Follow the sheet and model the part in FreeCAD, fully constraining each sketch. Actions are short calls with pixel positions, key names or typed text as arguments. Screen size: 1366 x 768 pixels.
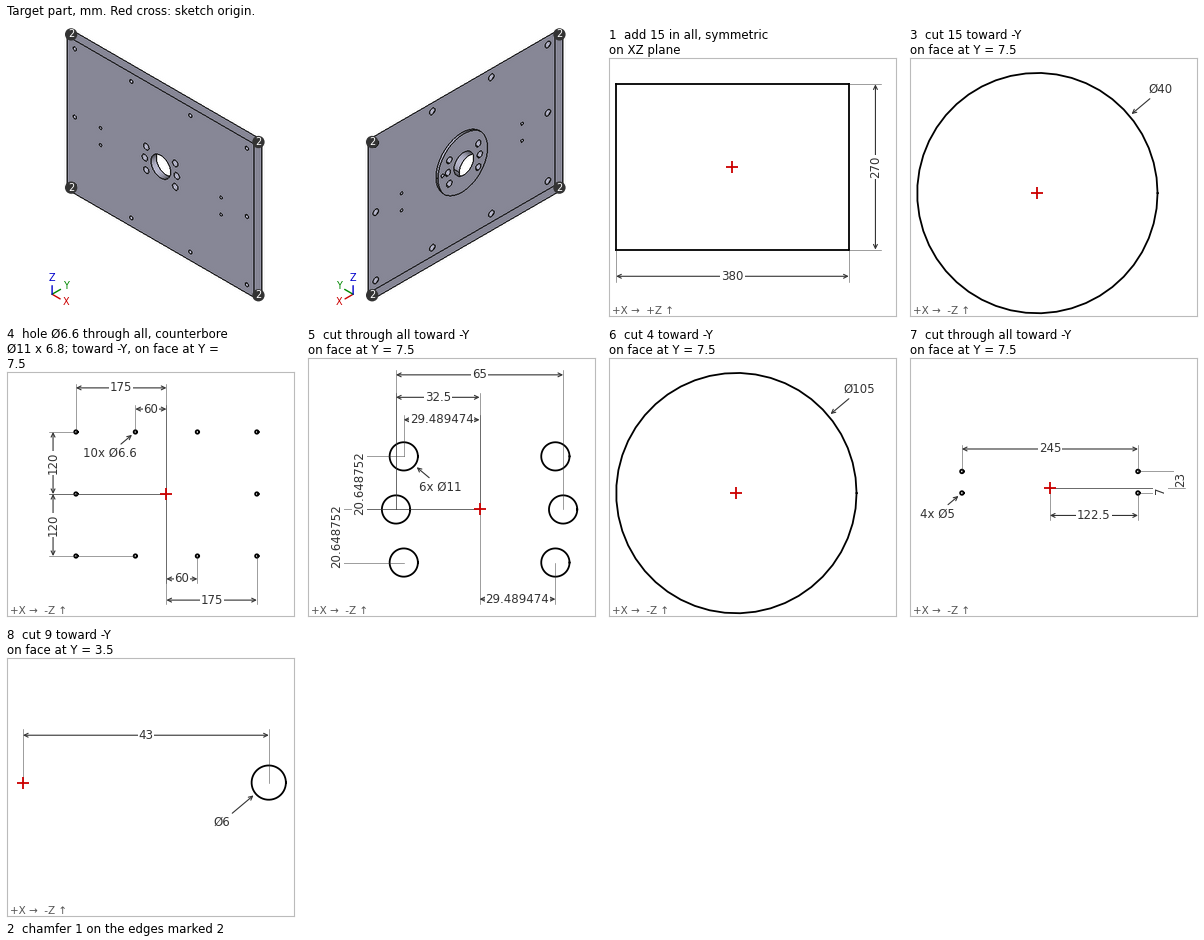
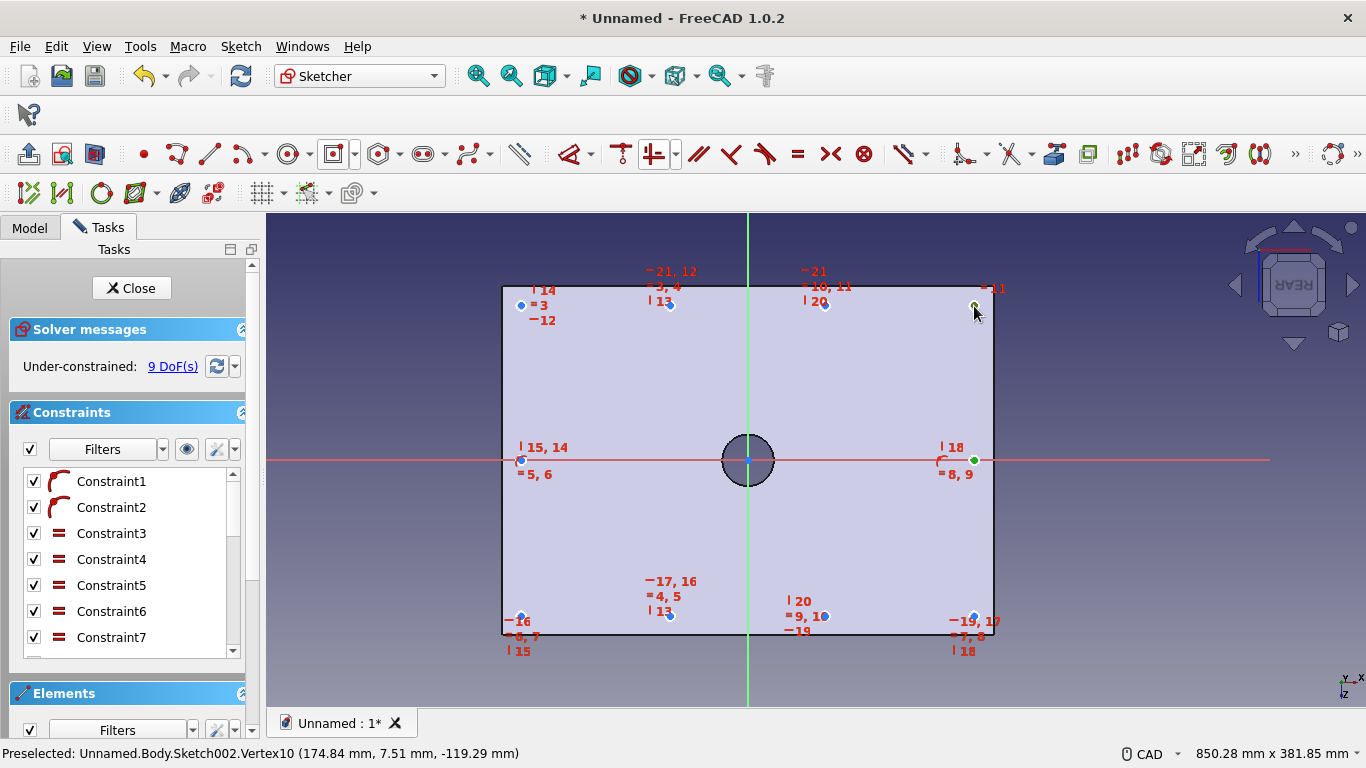
click(676, 154)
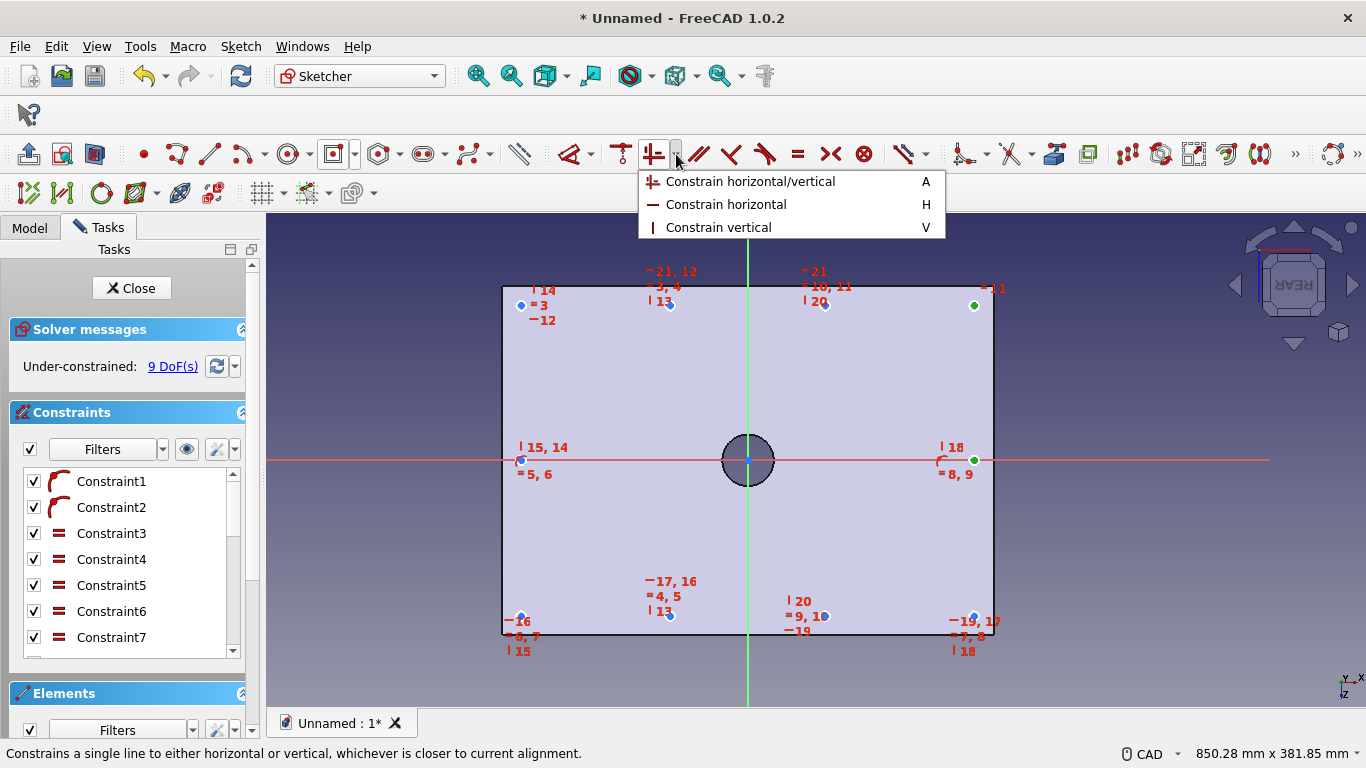
click(792, 228)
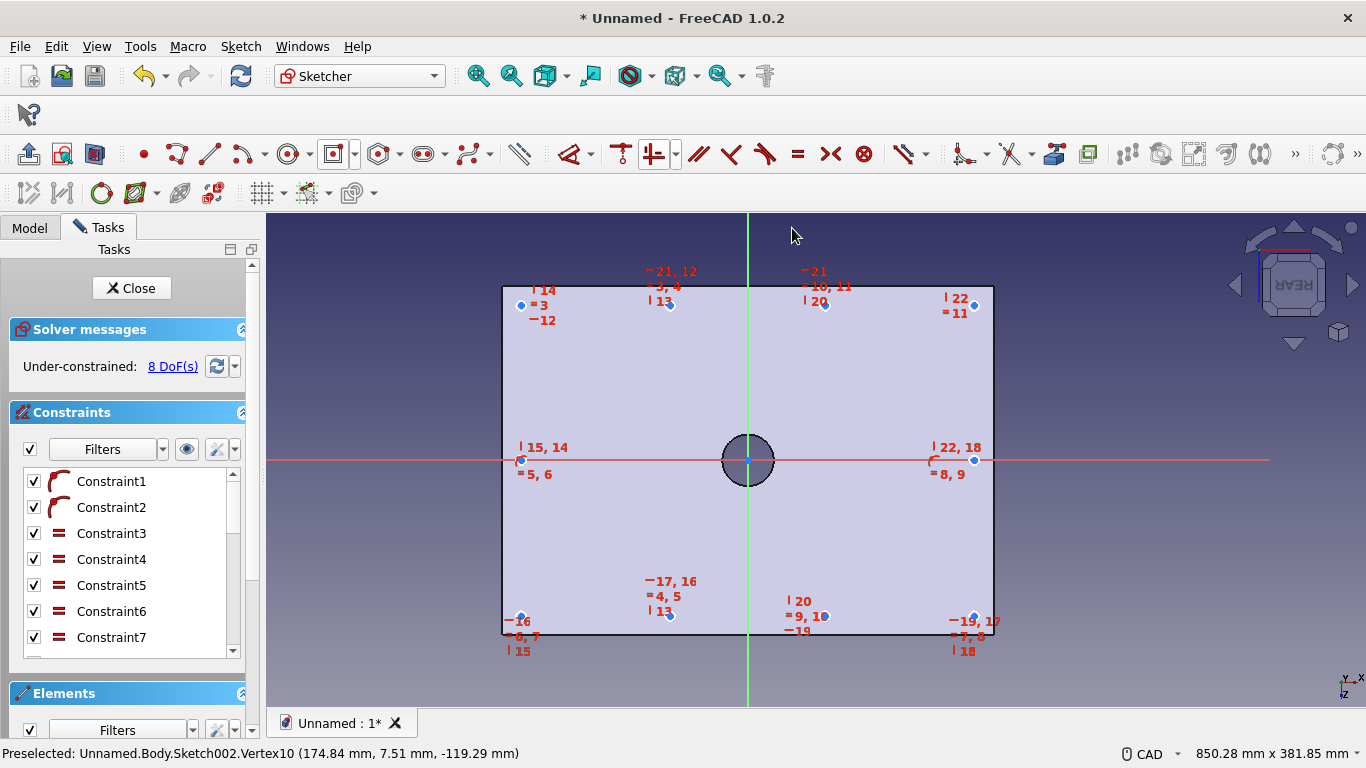
click(823, 308)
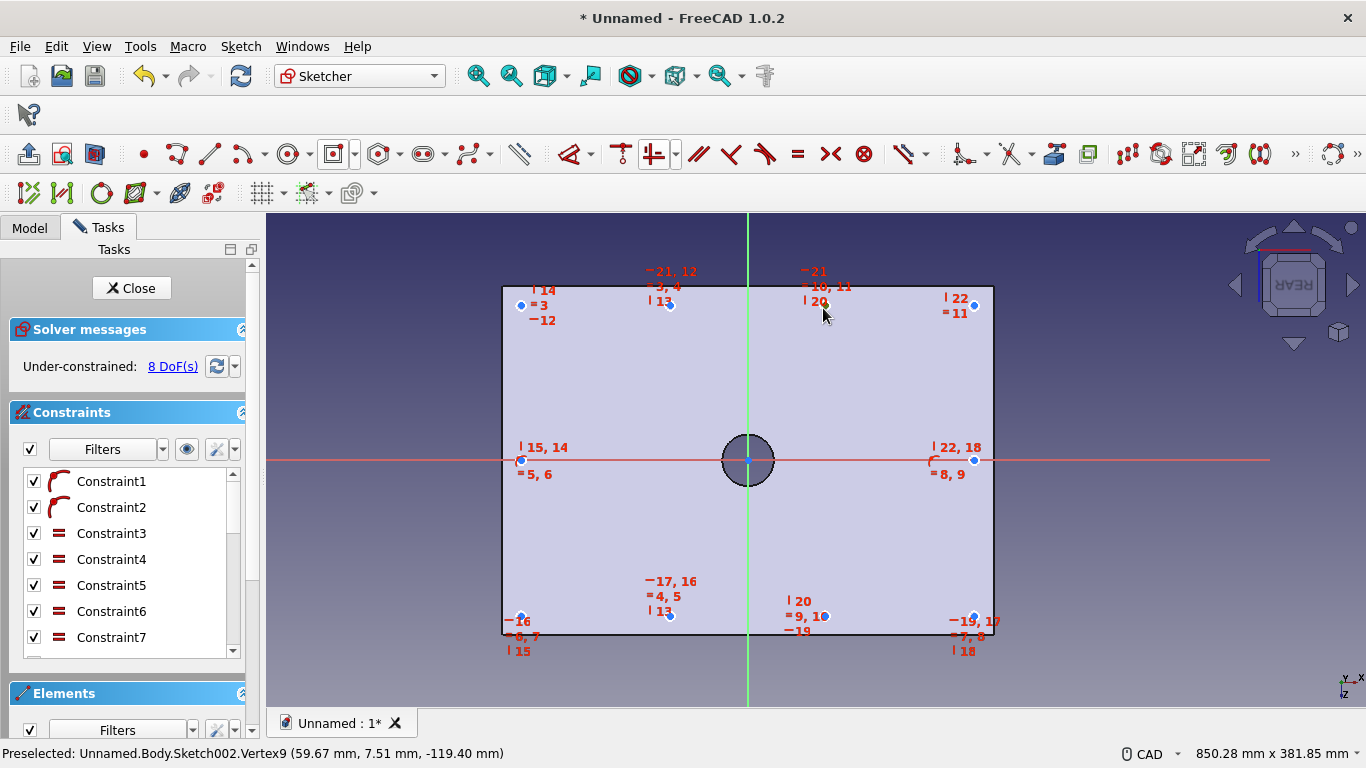
click(974, 306)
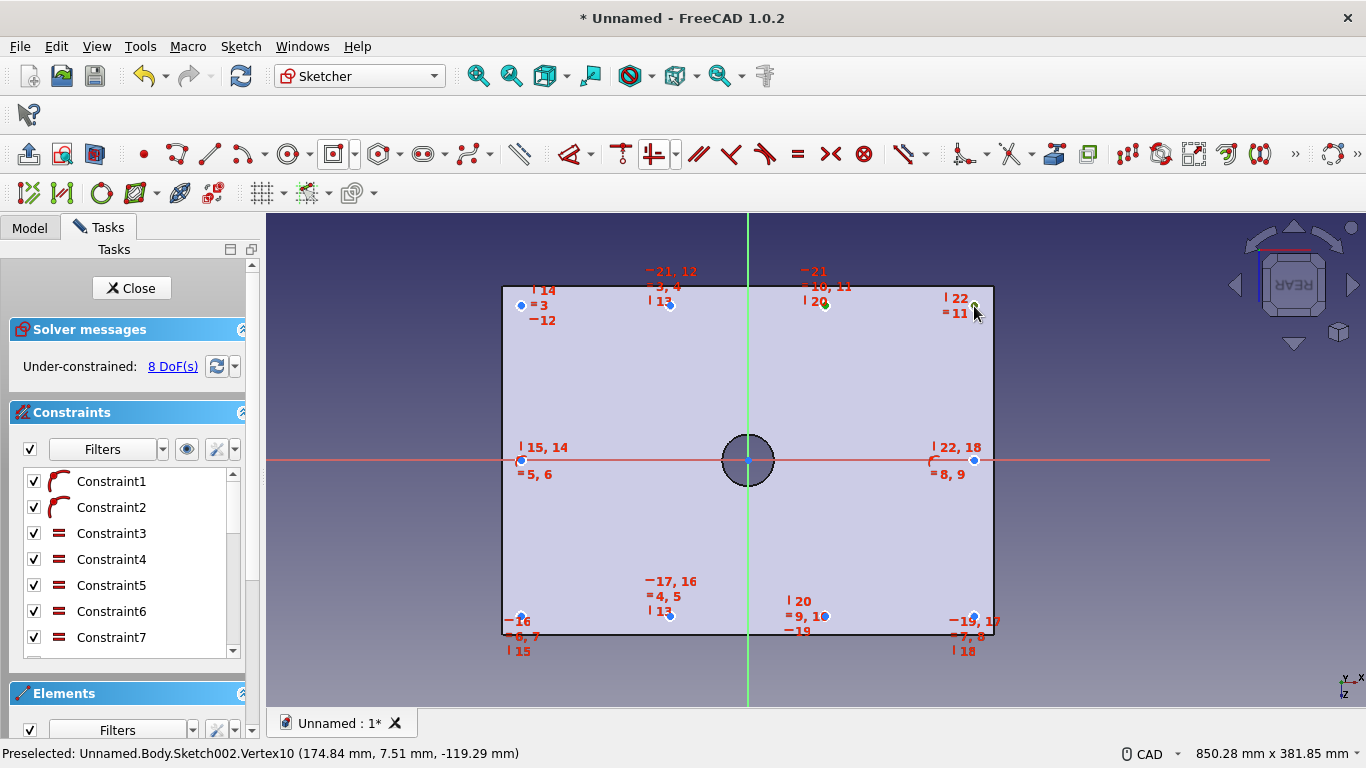
key(h)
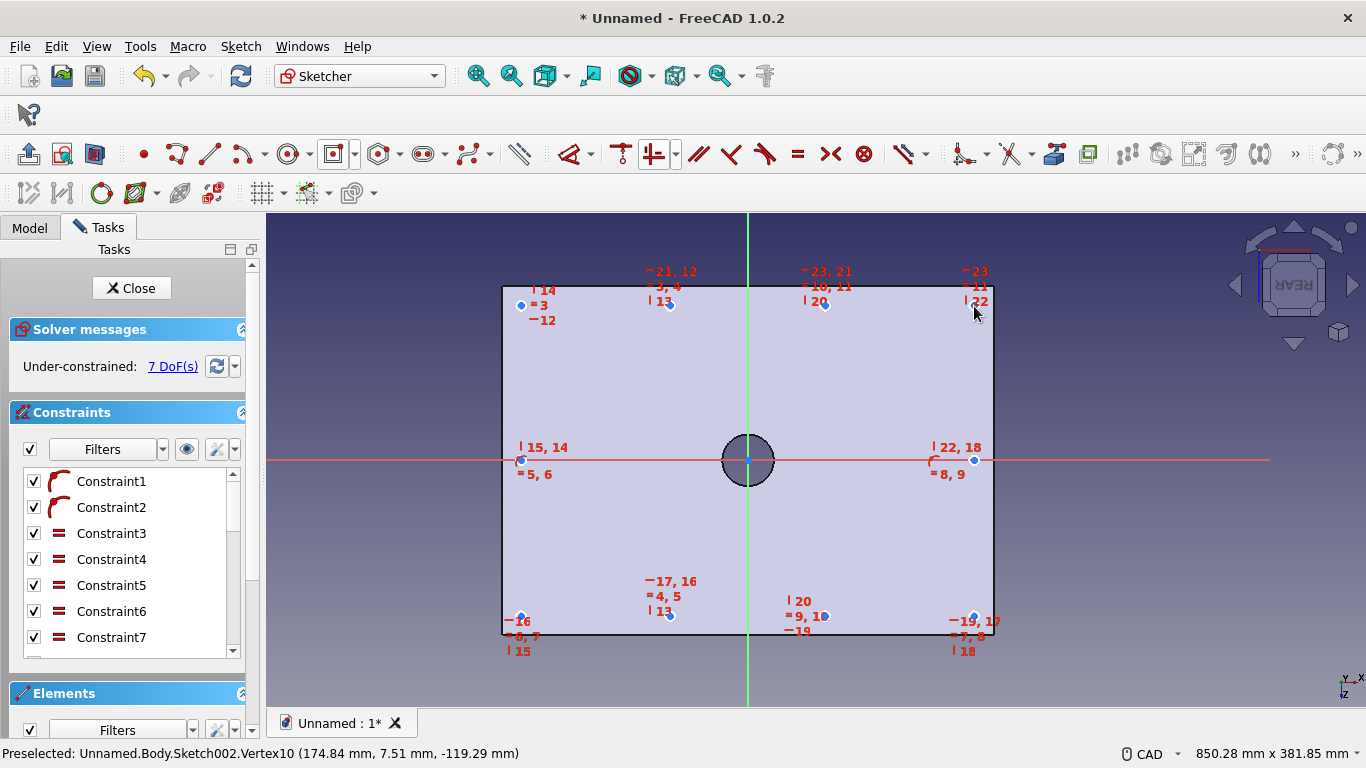
click(568, 154)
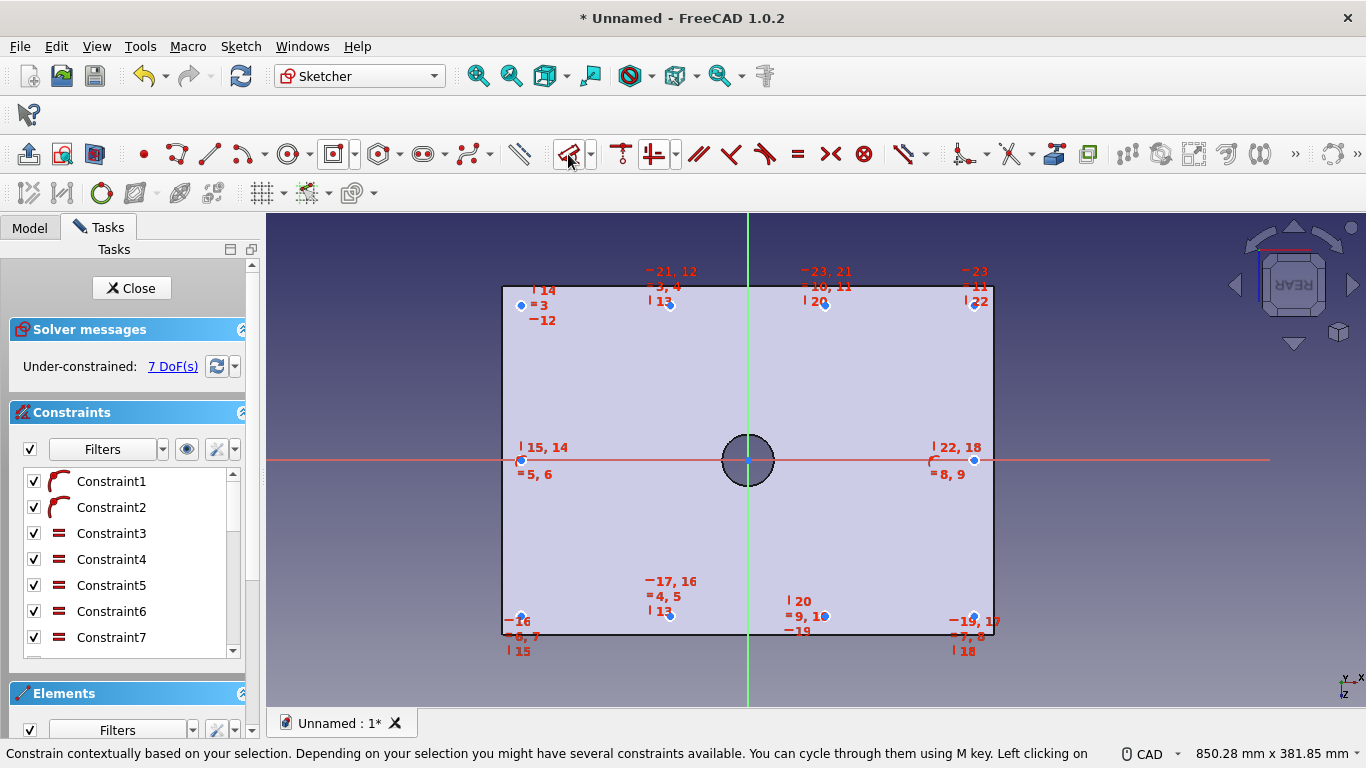
scroll(518, 302, up, 8)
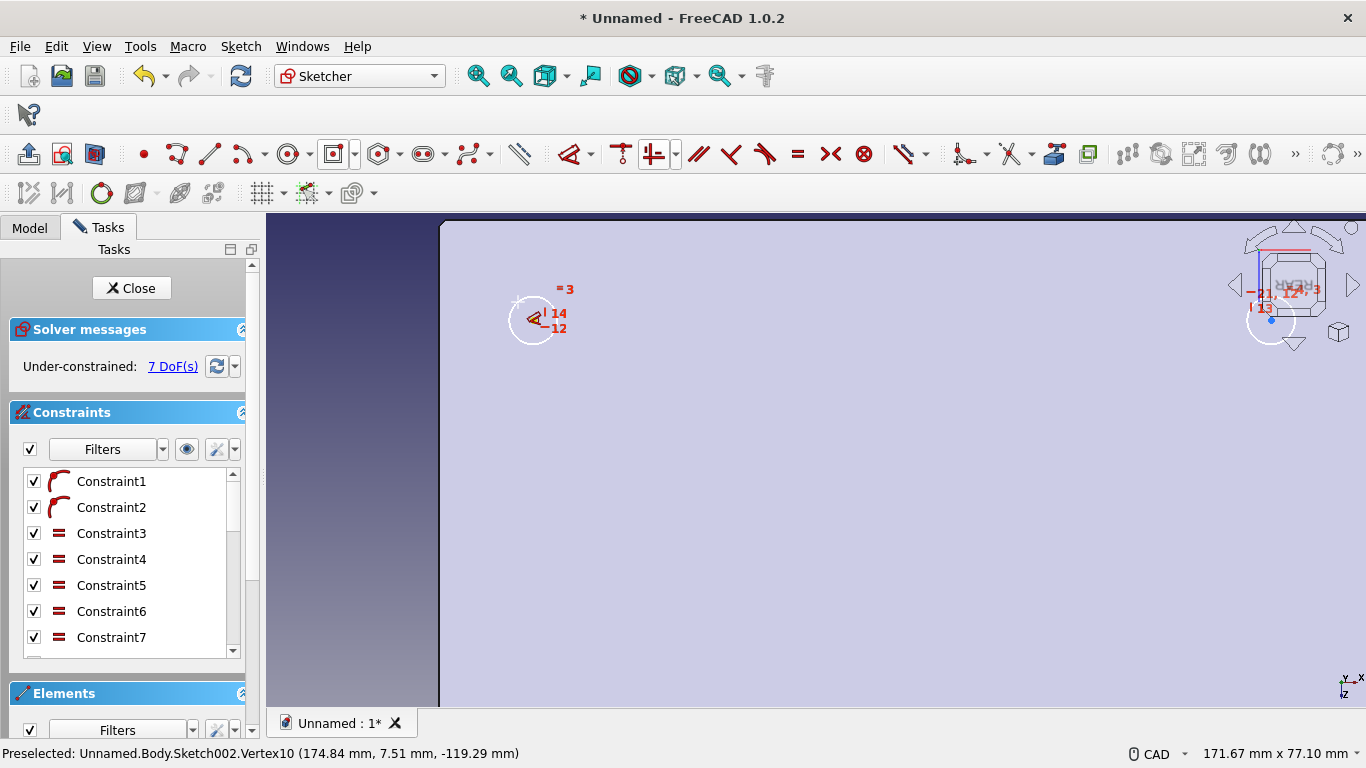
click(516, 304)
click(493, 282)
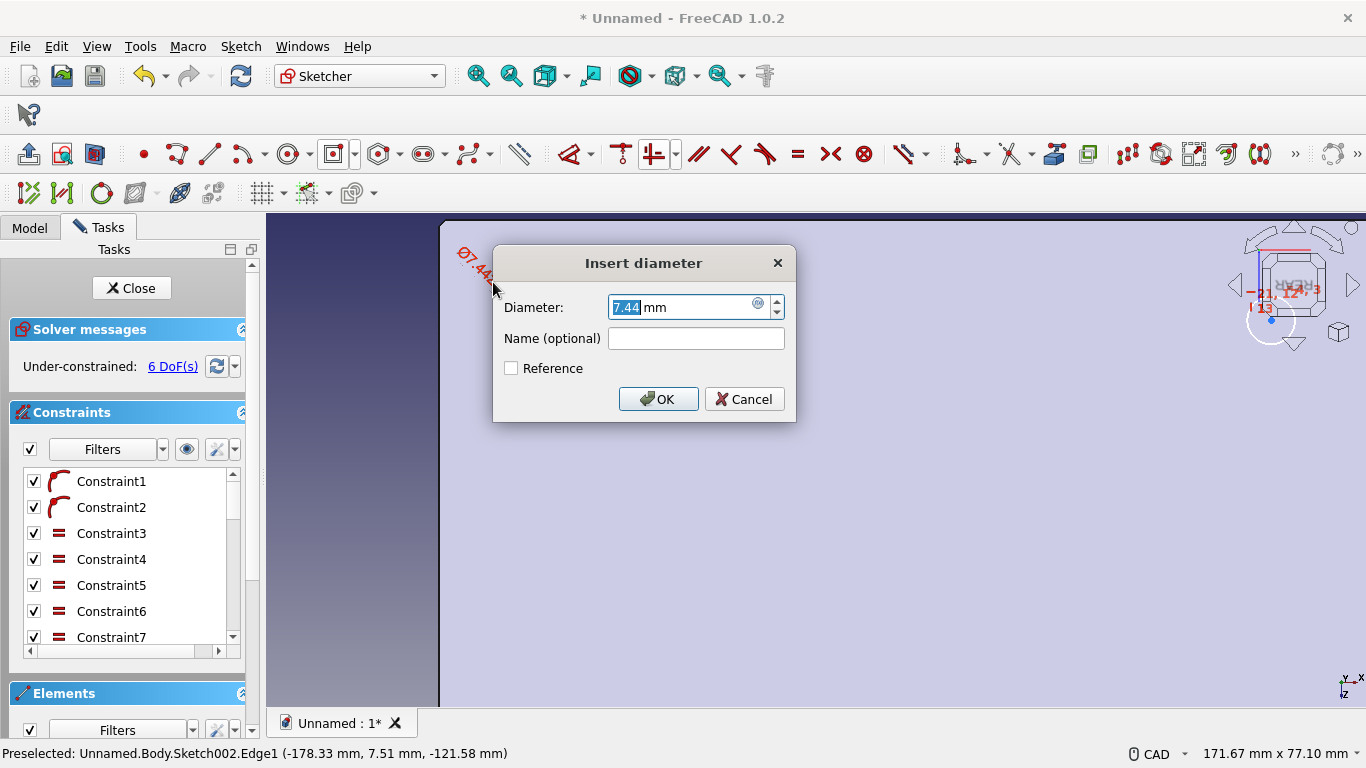
text(6.6)
key(Return)